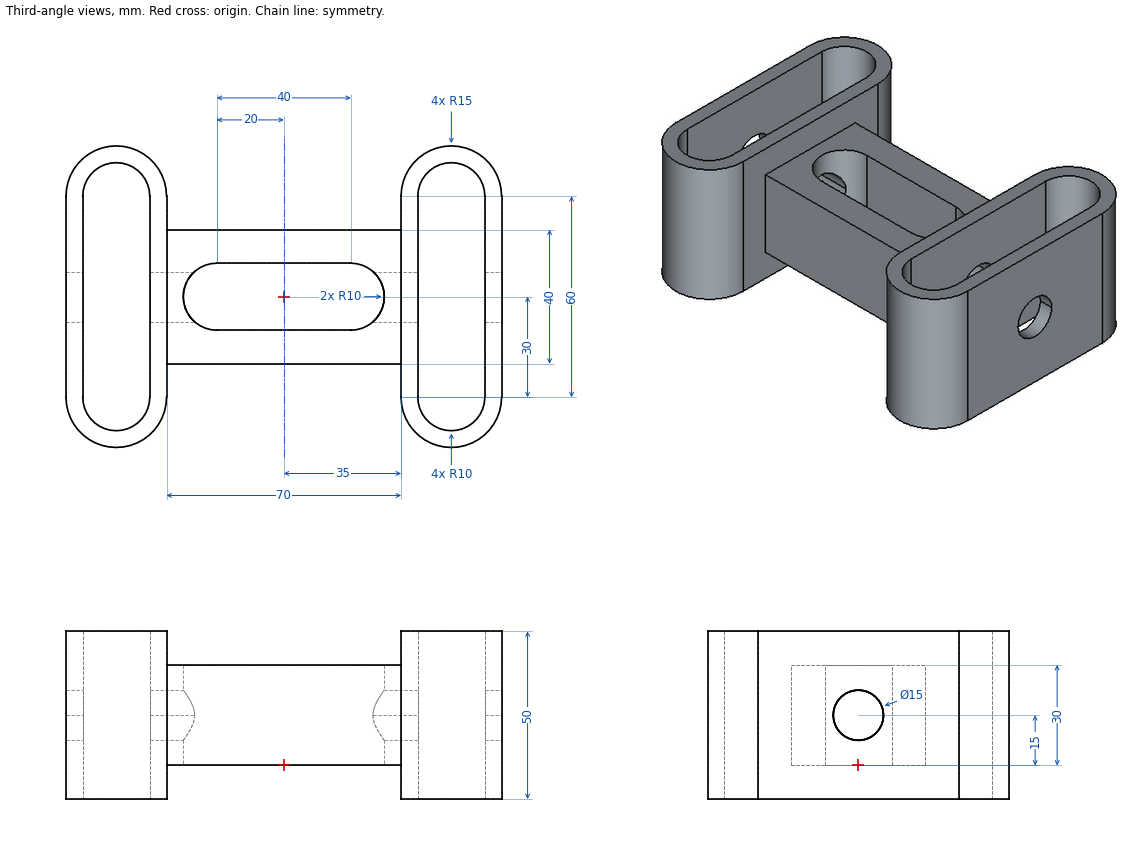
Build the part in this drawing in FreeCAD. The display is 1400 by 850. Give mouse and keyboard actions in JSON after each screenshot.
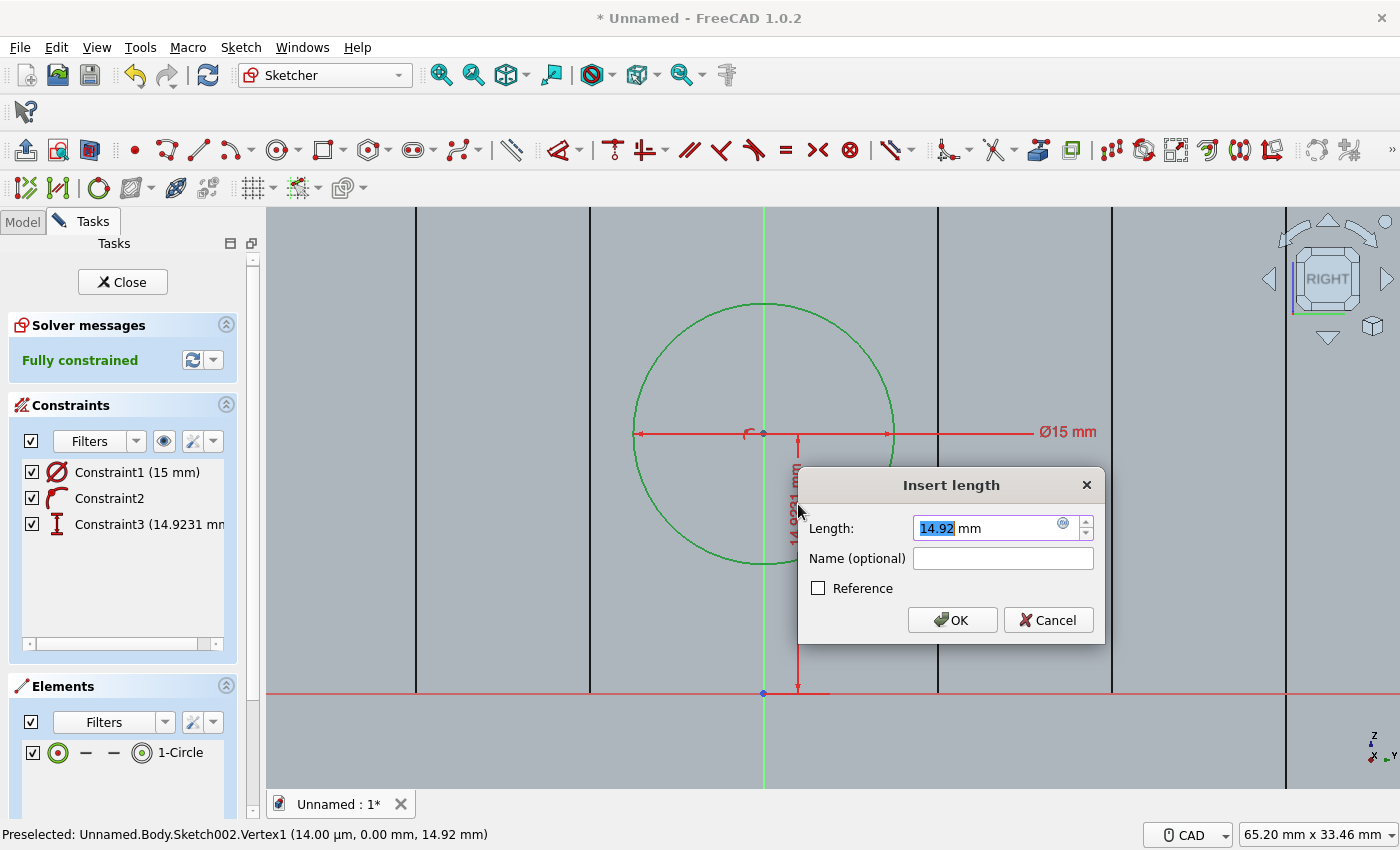
{"action": "type", "text": "15"}
{"action": "key", "text": "Return"}
{"action": "key", "text": "Escape"}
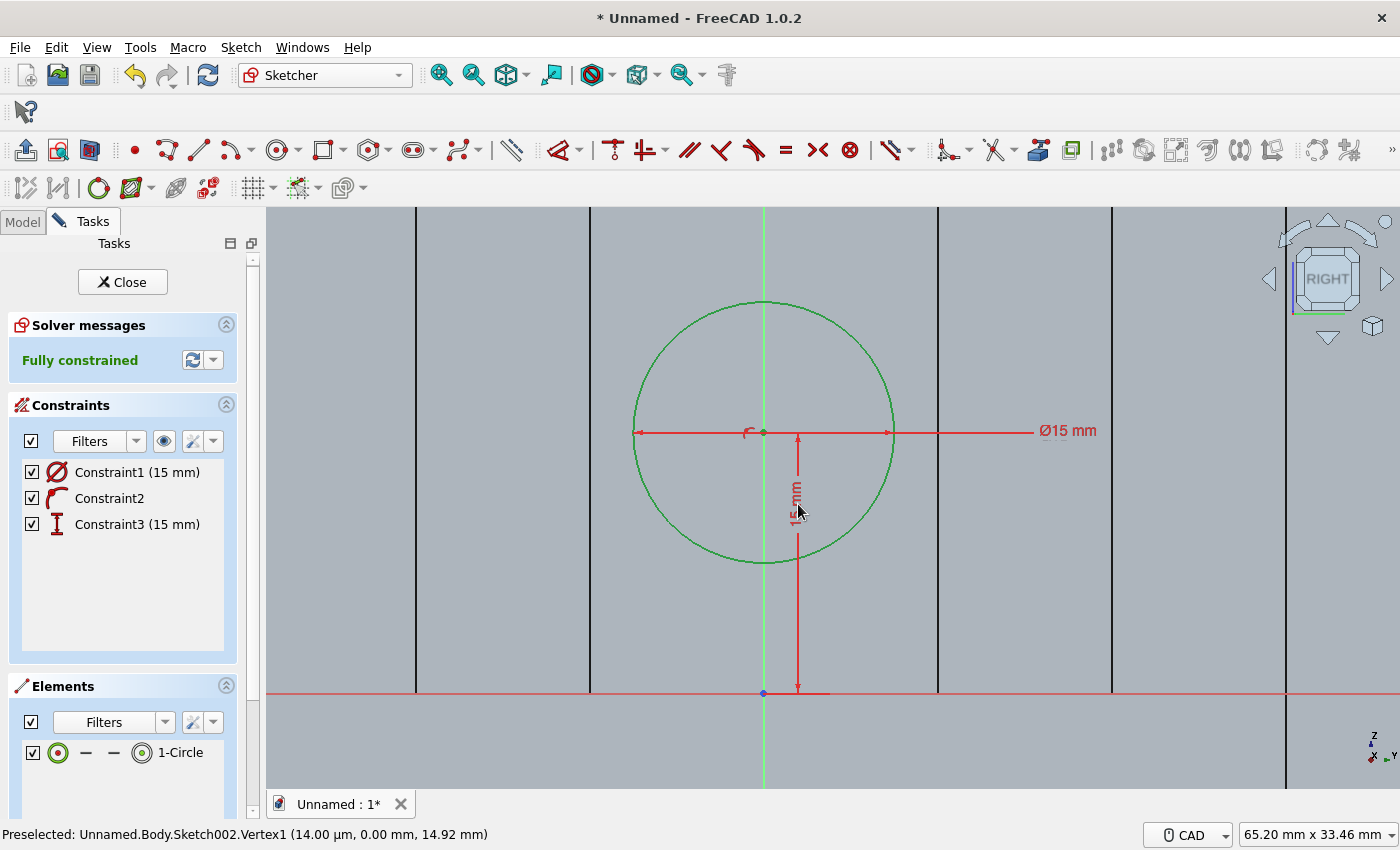
{"action": "left_click", "coordinate": [123, 282]}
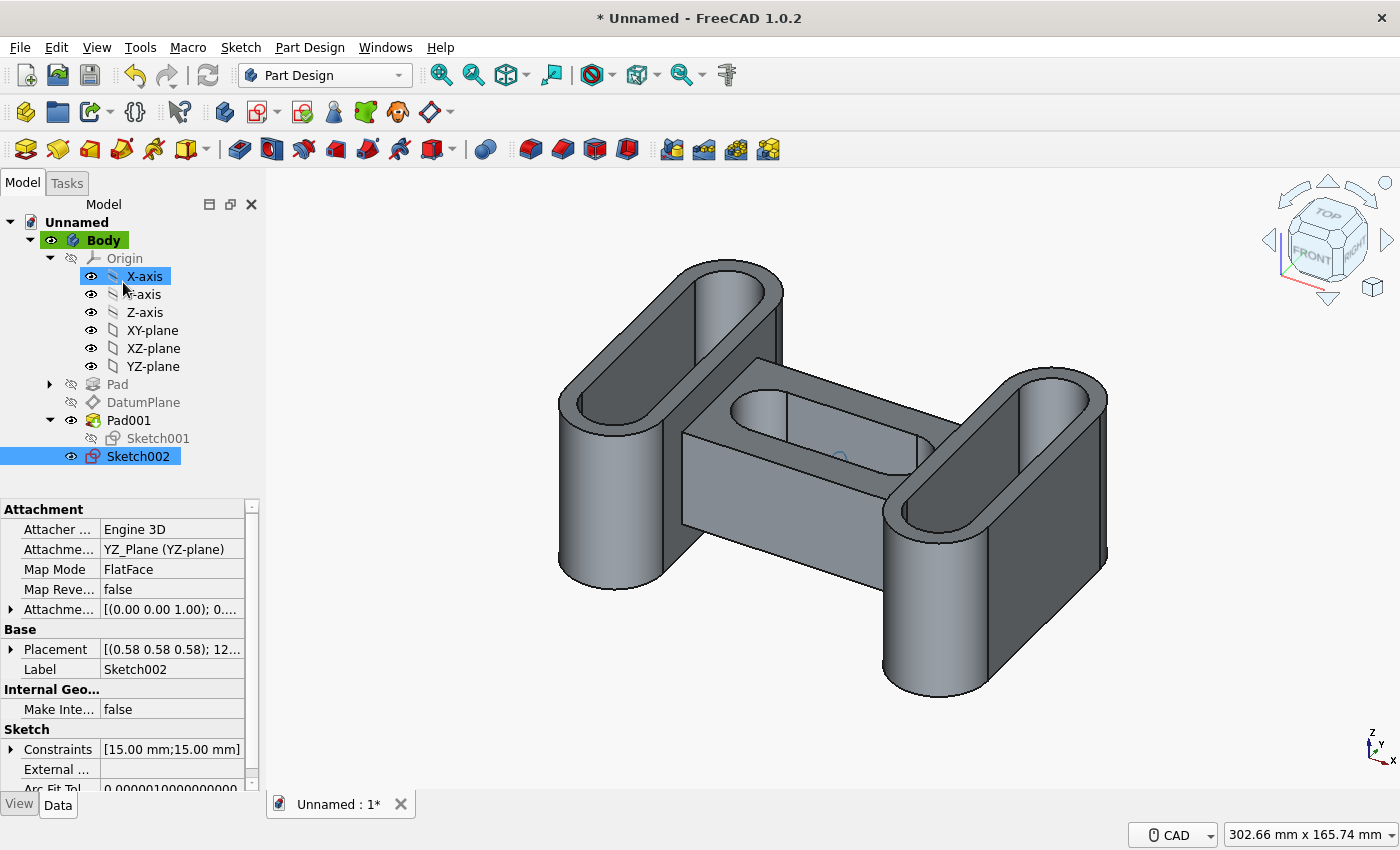
{"action": "left_click", "coordinate": [240, 150]}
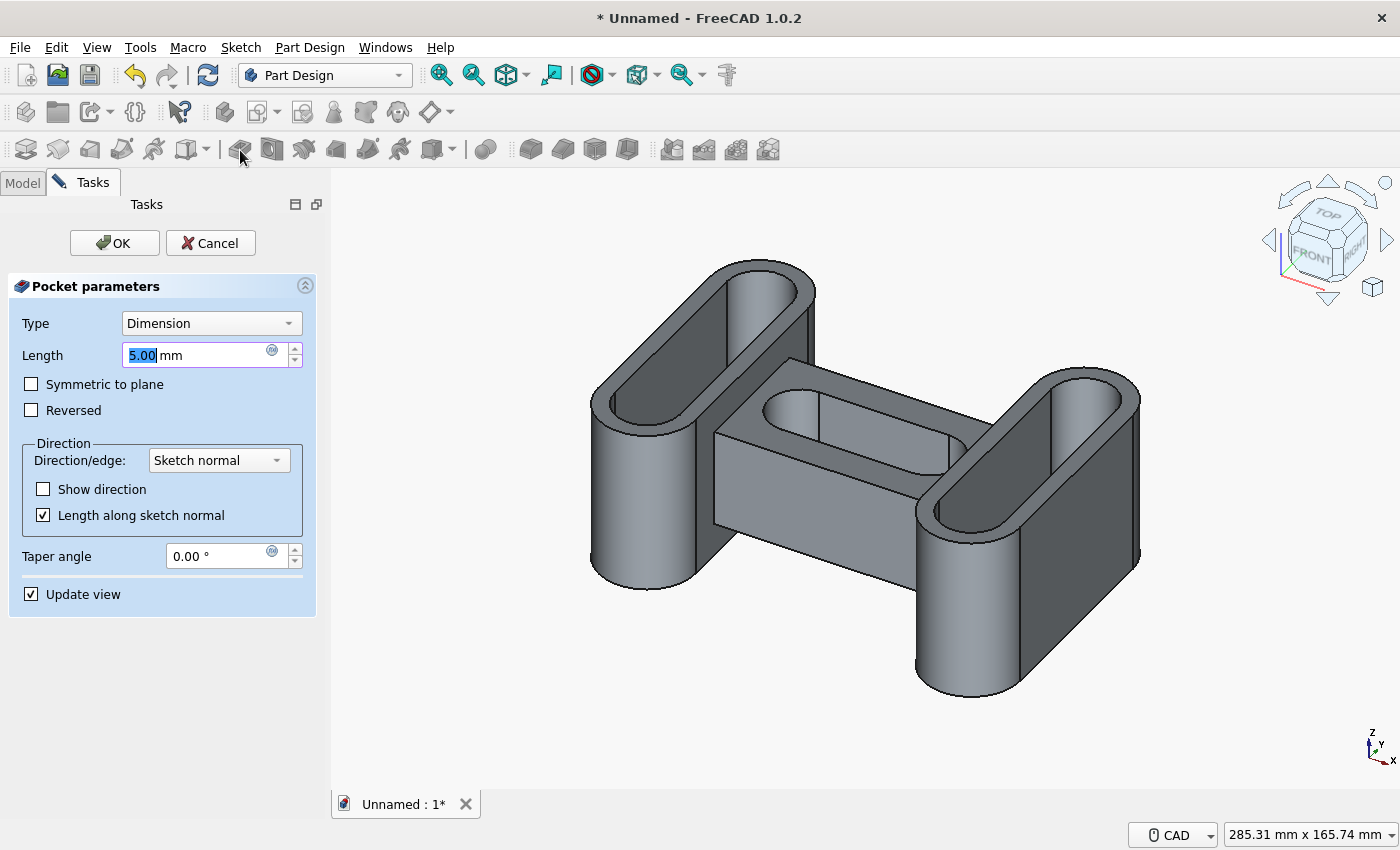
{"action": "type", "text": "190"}
{"action": "key", "text": "Tab"}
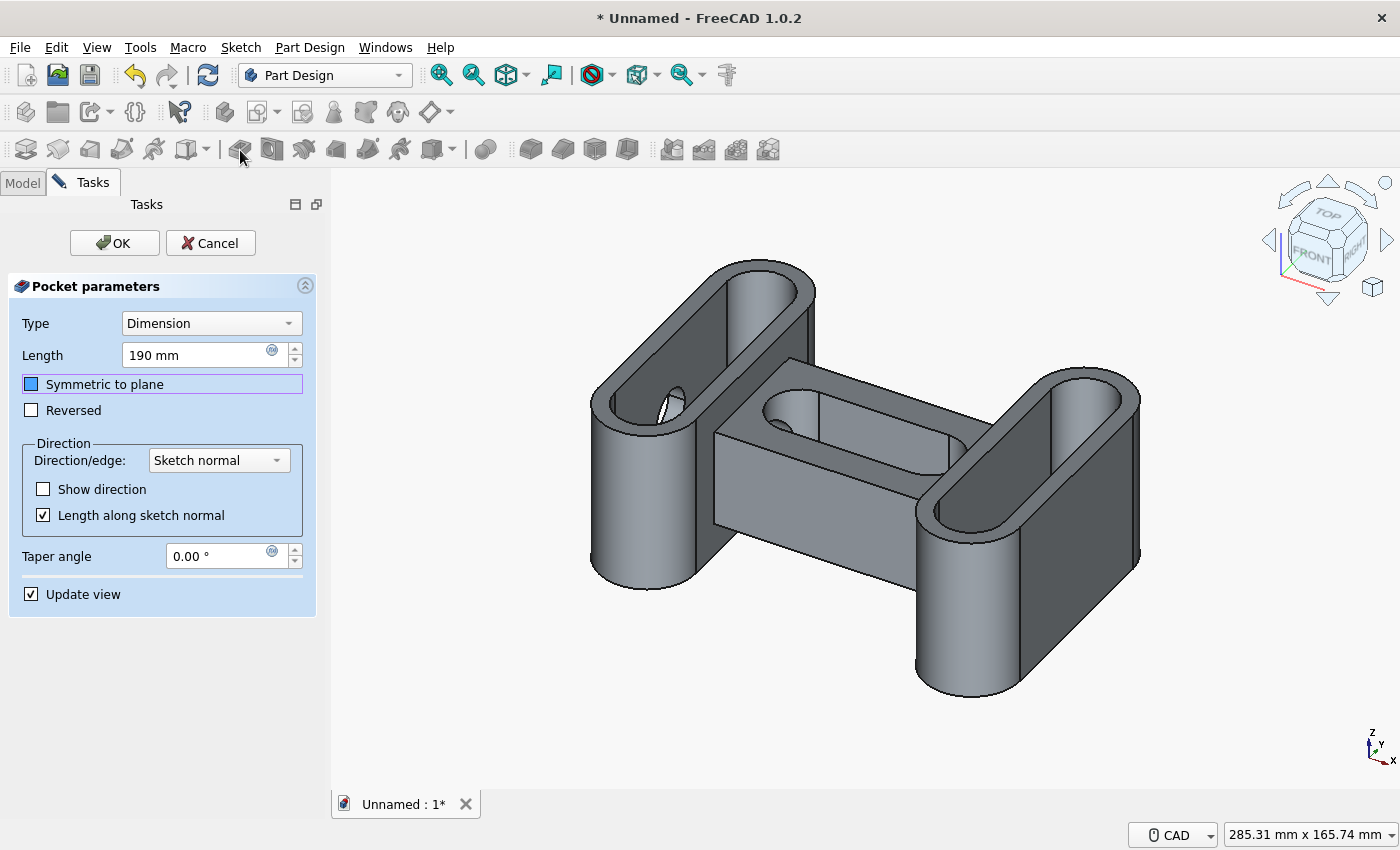
{"action": "left_click", "coordinate": [30, 384]}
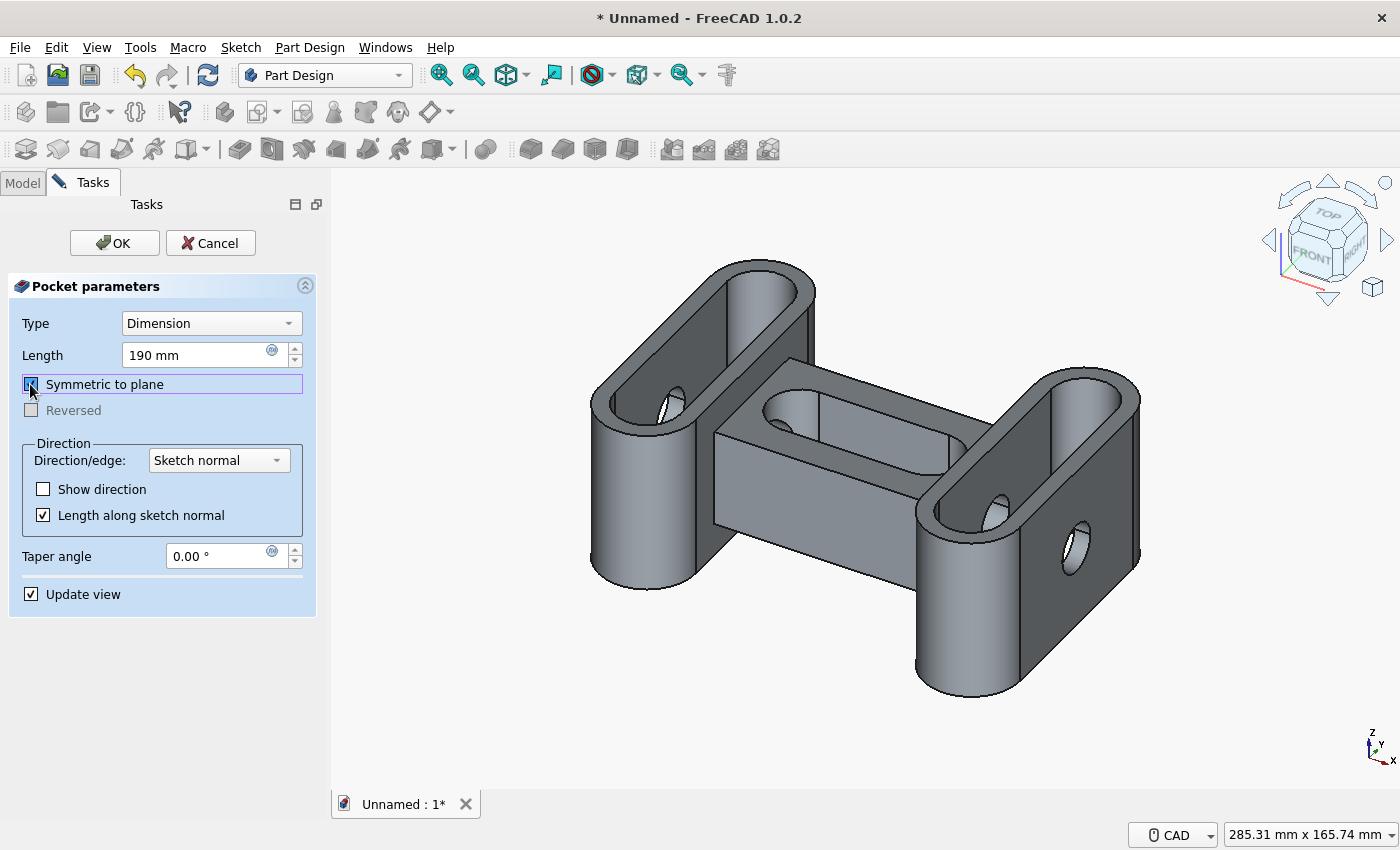
{"action": "left_click", "coordinate": [115, 243]}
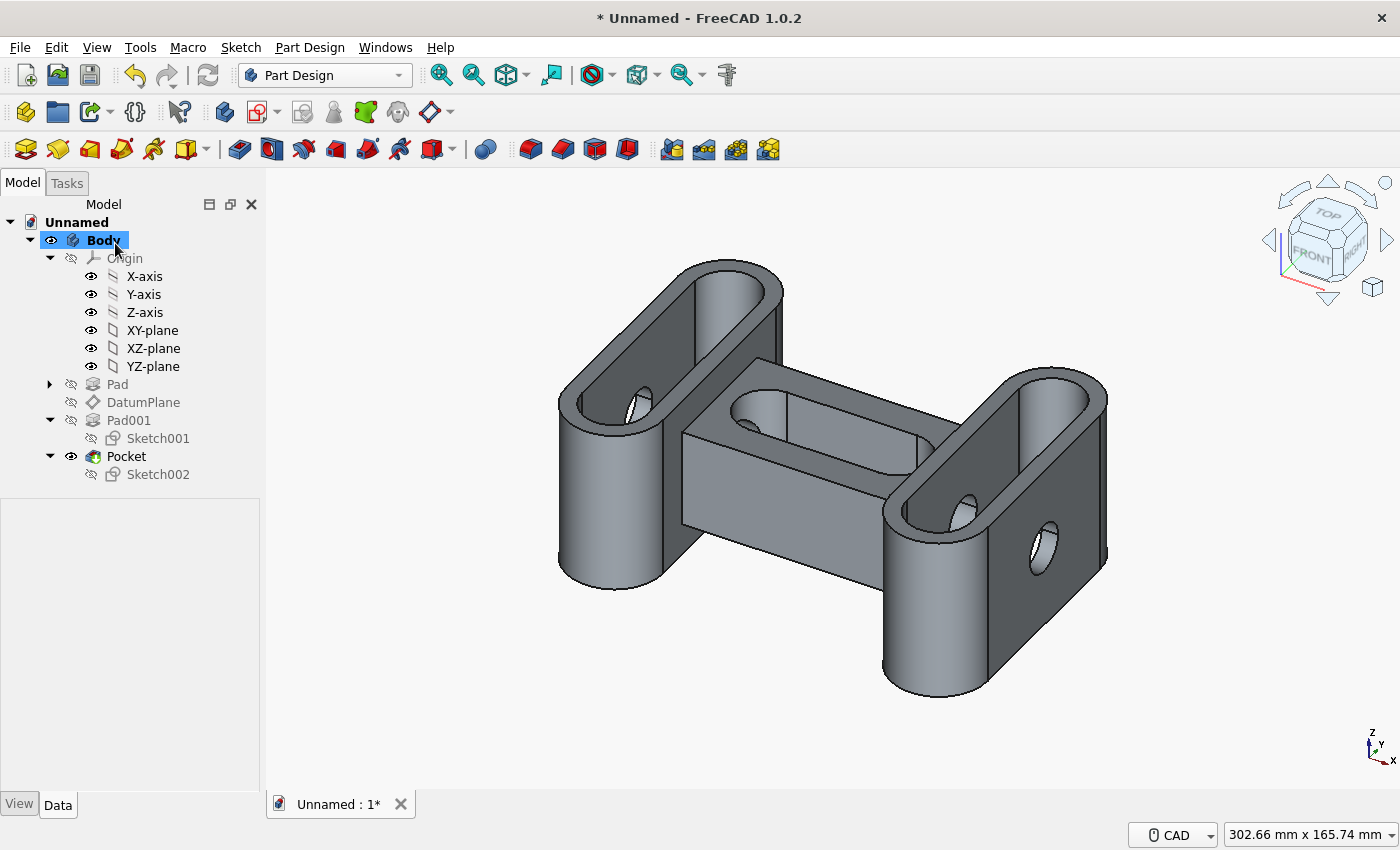
{"action": "key", "text": "0"}